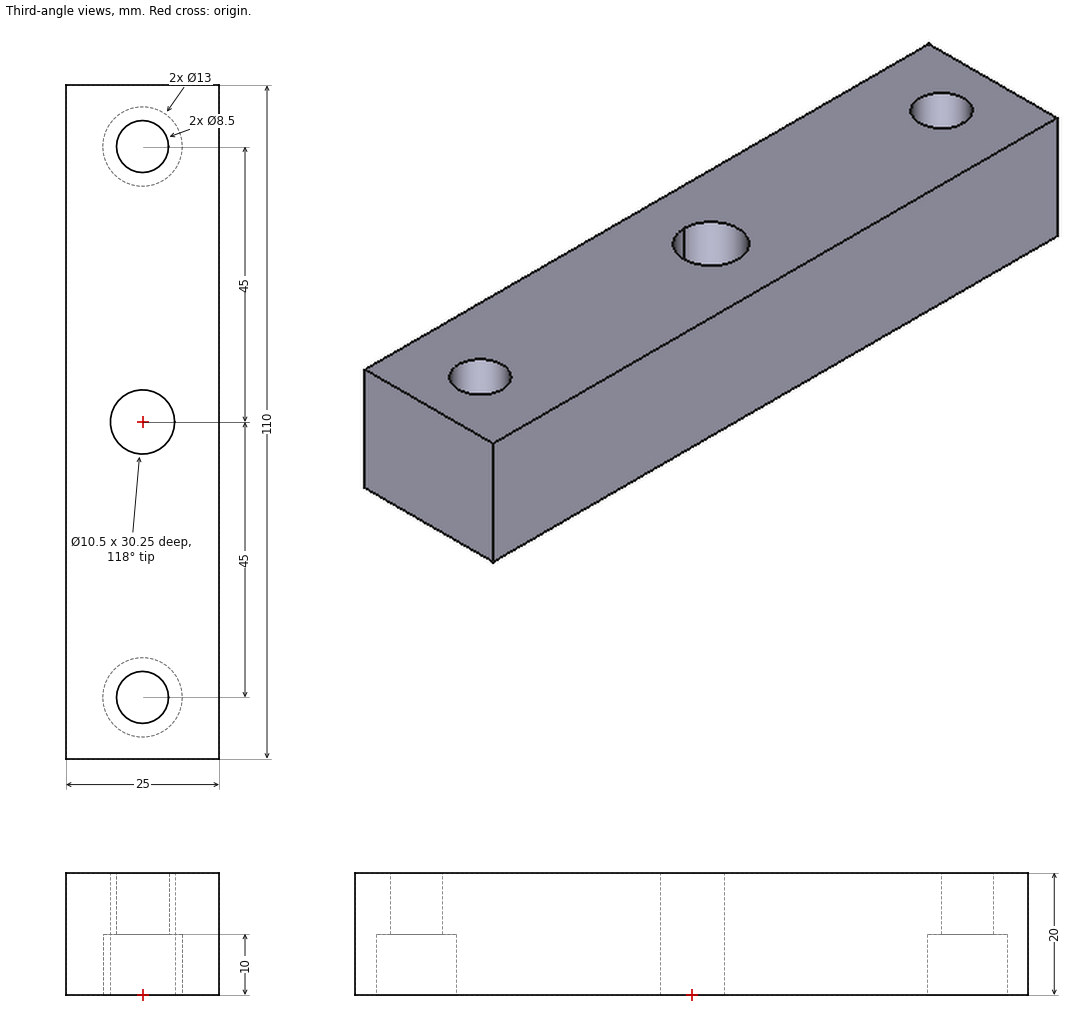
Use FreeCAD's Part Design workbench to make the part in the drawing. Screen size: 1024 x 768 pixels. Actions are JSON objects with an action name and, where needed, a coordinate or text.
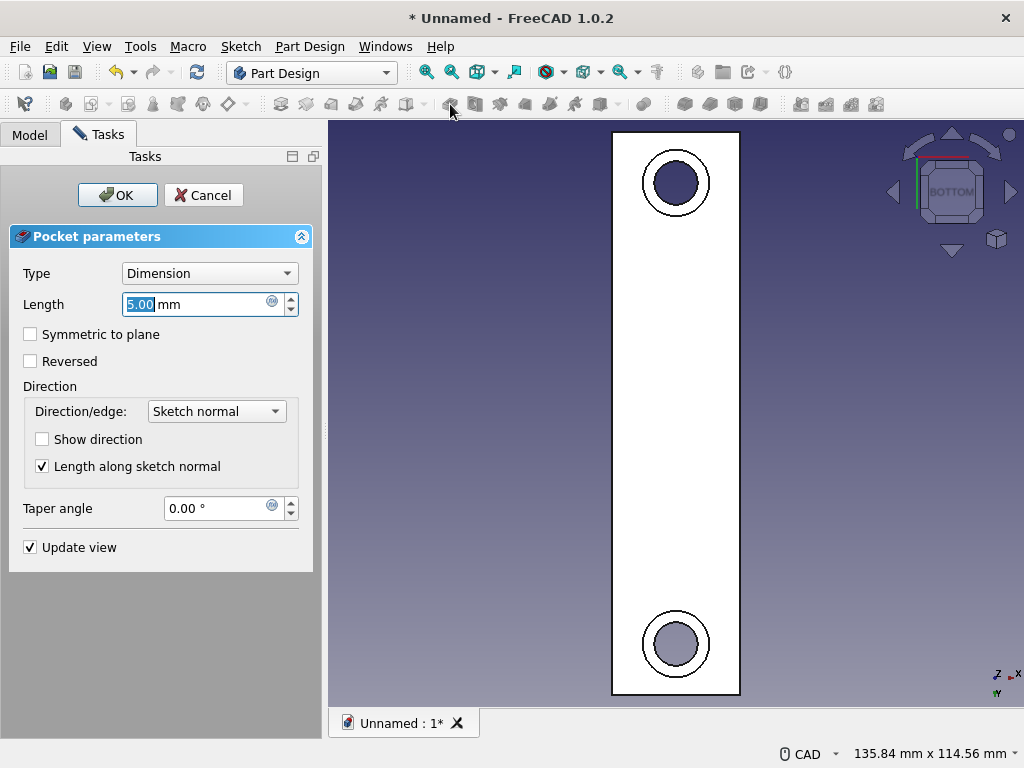
{"action": "type", "text": "10"}
{"action": "key", "text": "Tab"}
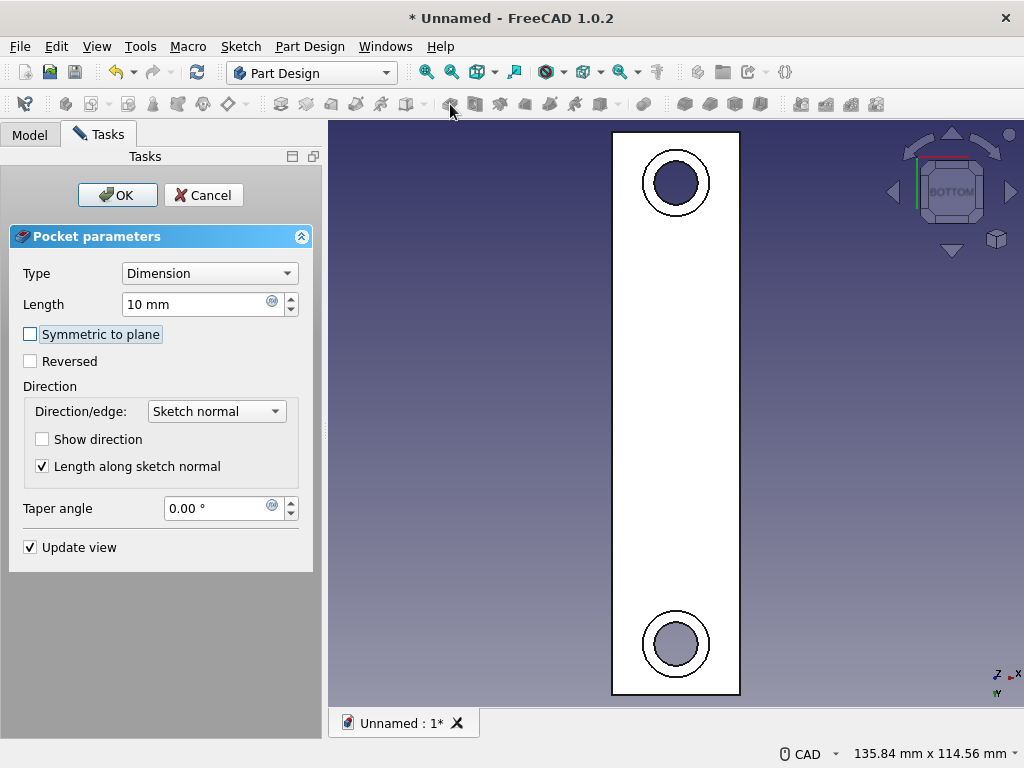
{"action": "left_click", "coordinate": [118, 195]}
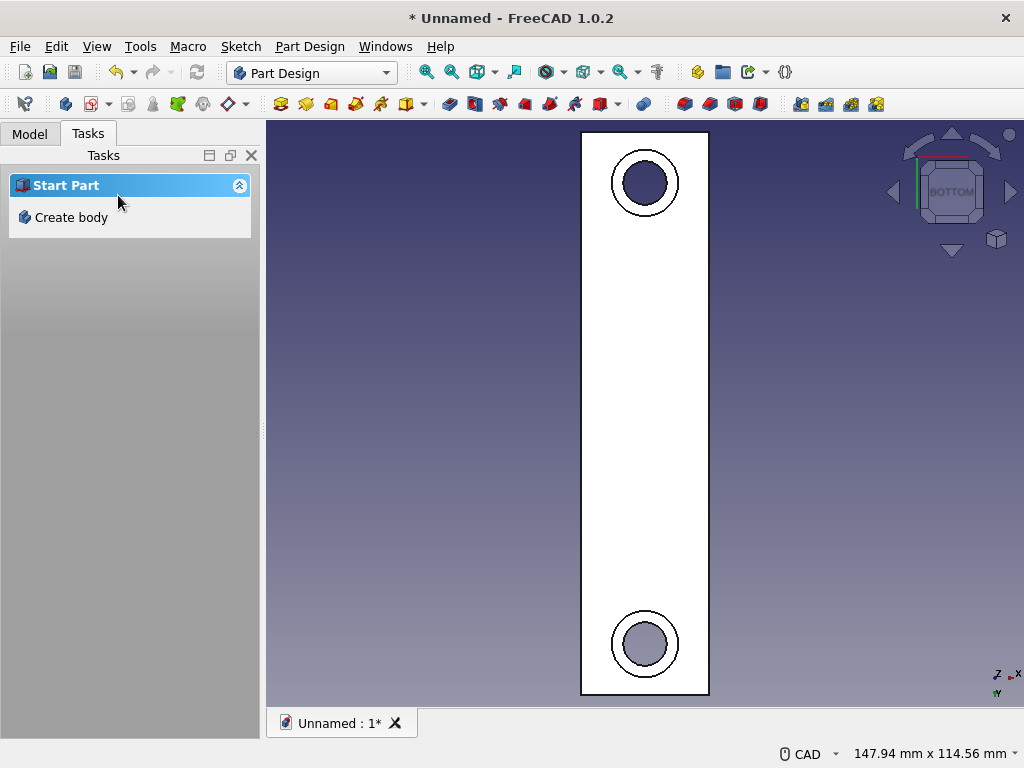
{"action": "left_click", "coordinate": [90, 104]}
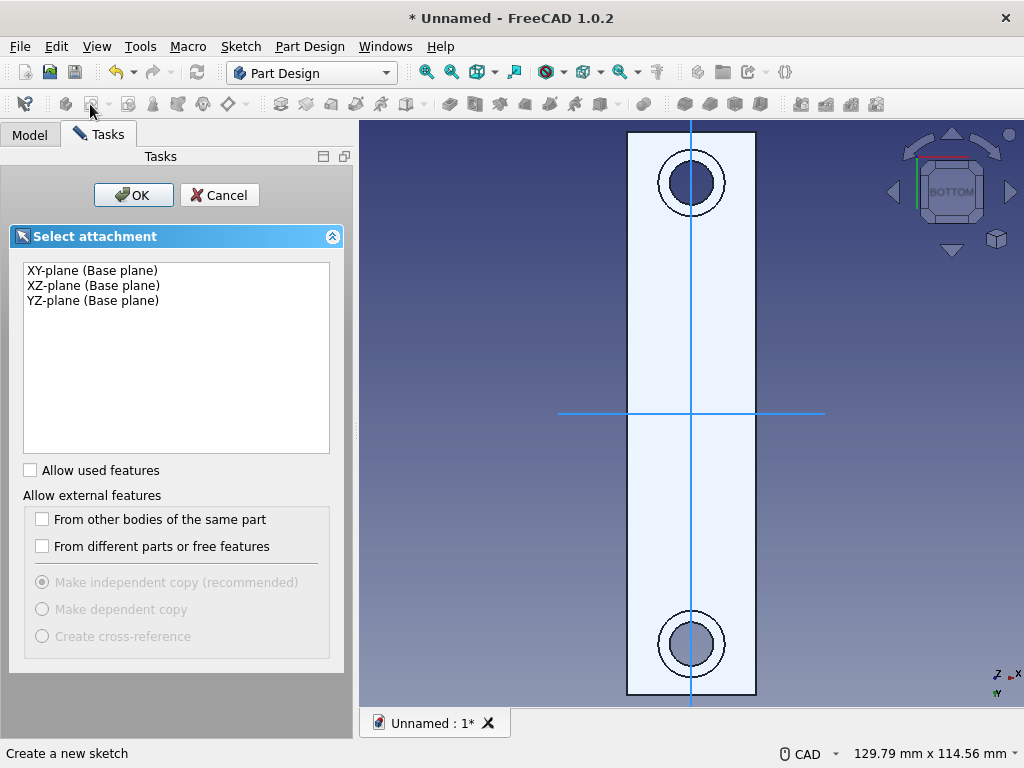
{"action": "left_click", "coordinate": [84, 270]}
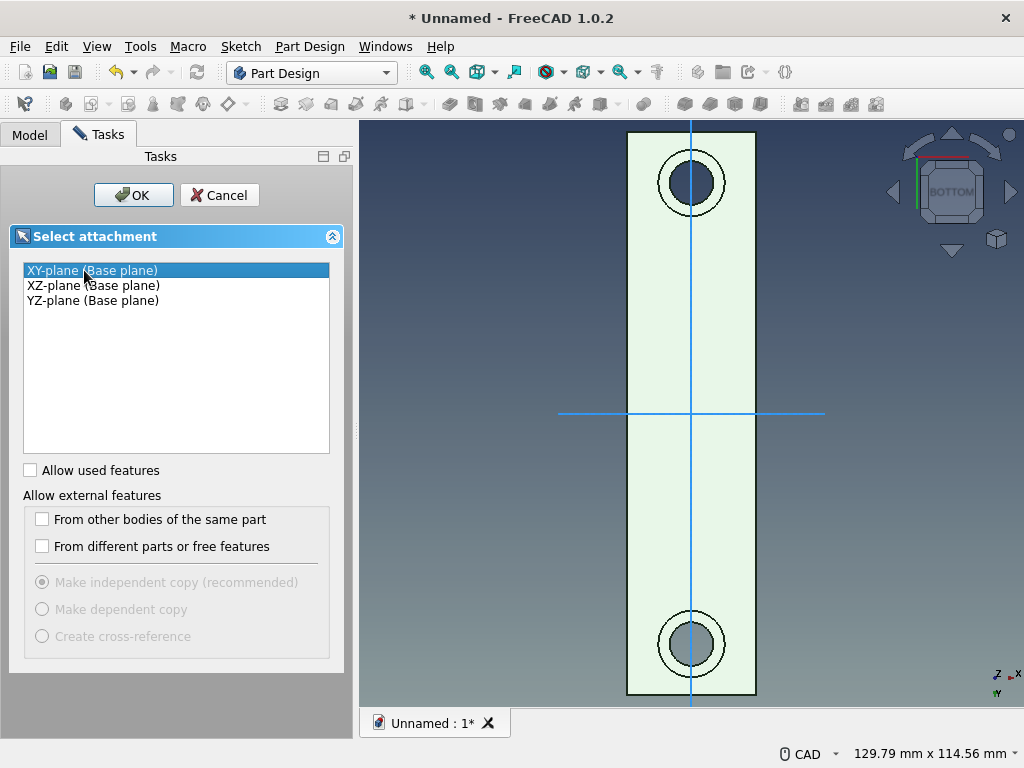
{"action": "left_click", "coordinate": [134, 195]}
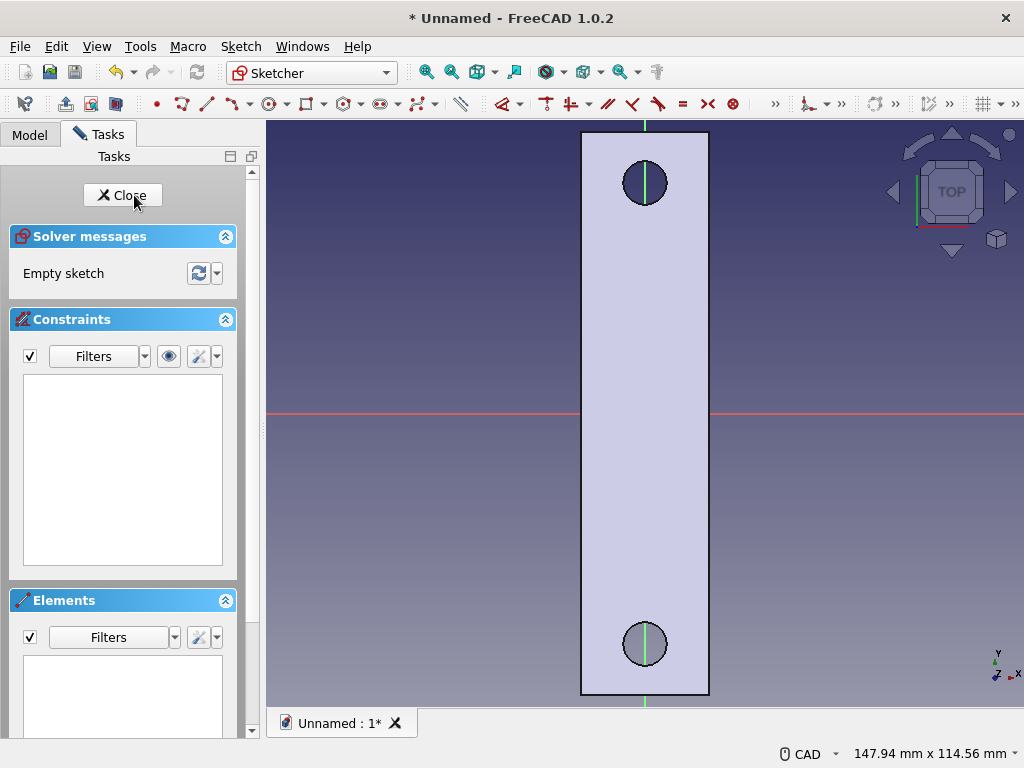
{"action": "key", "text": "q s"}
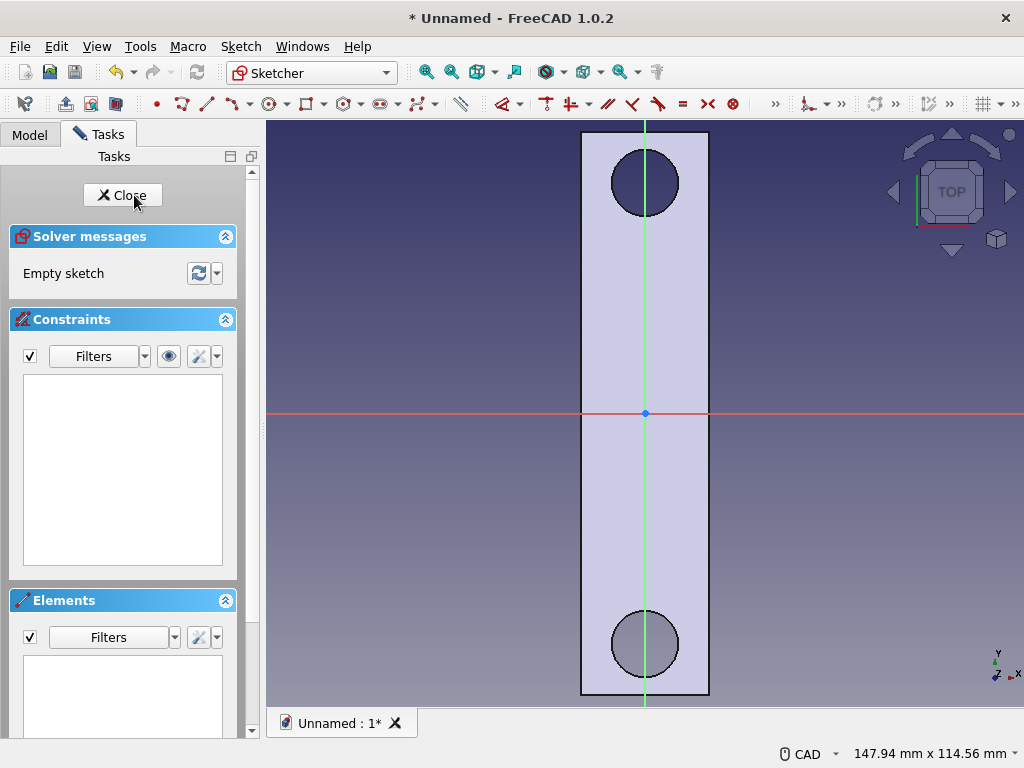
{"action": "scroll", "coordinate": [656, 413], "scroll_direction": "up", "scroll_amount": 10}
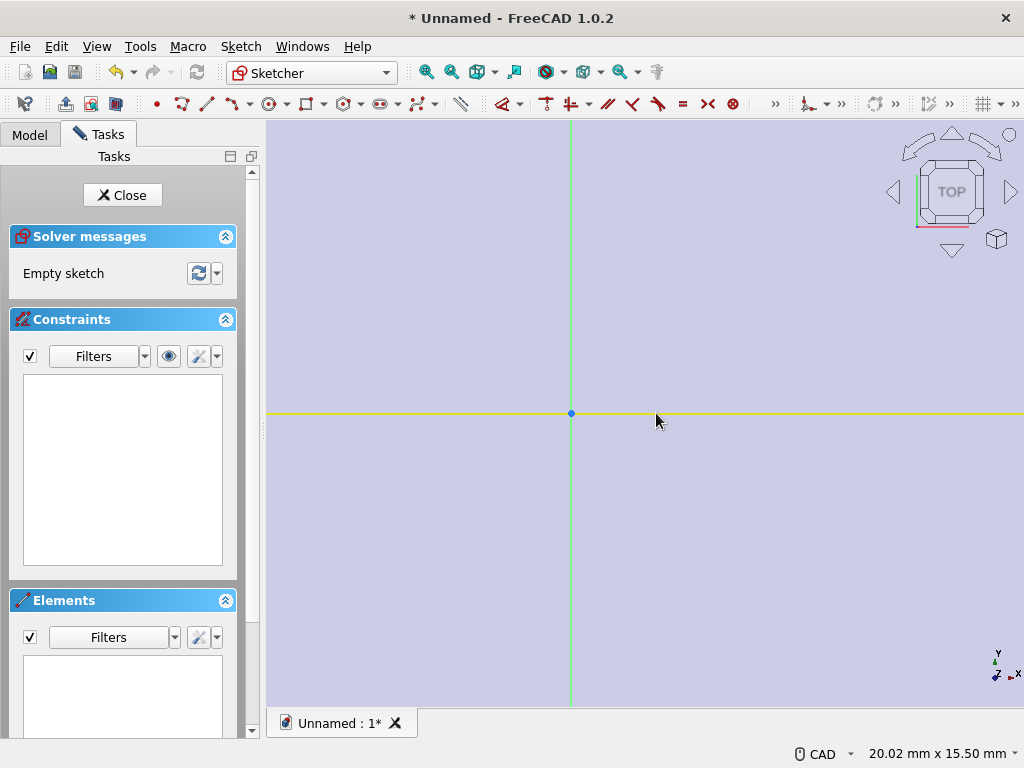
{"action": "left_click", "coordinate": [268, 104]}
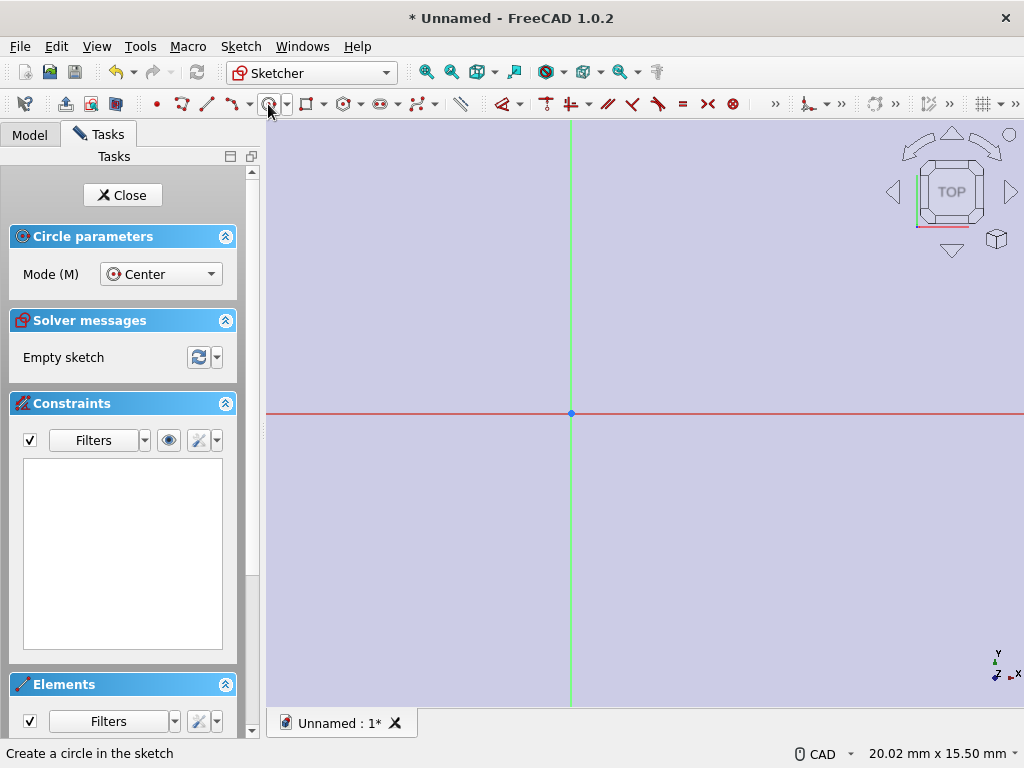
{"action": "left_click", "coordinate": [571, 413]}
{"action": "left_click", "coordinate": [712, 273]}
{"action": "key", "text": "Escape"}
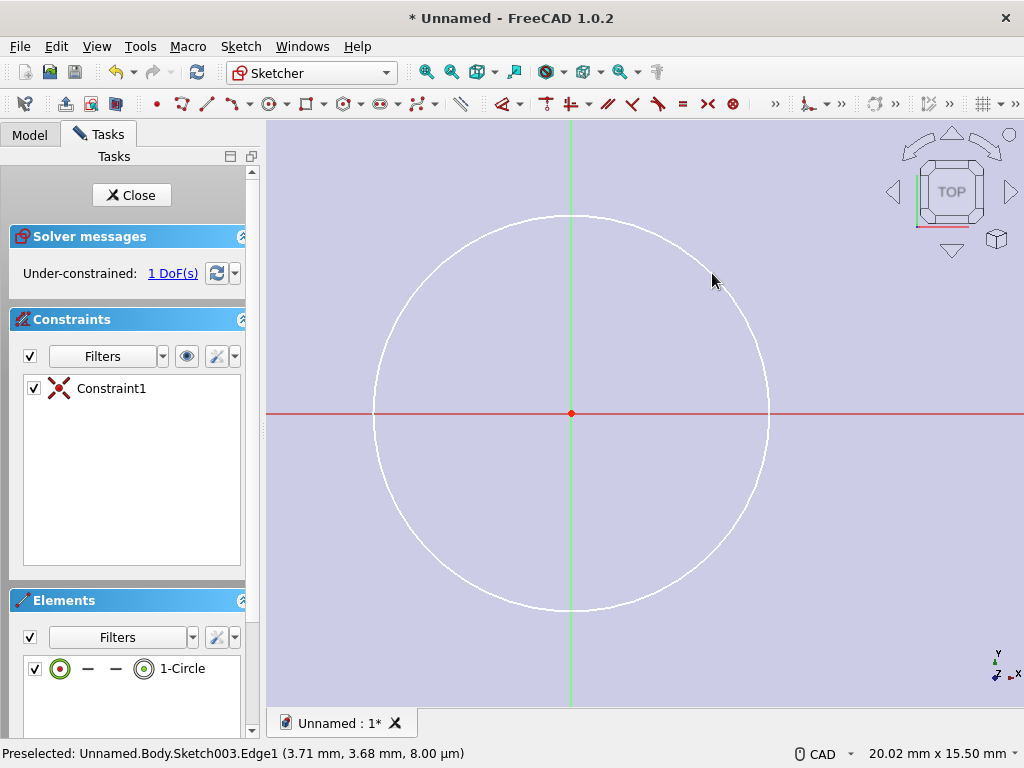
{"action": "left_click", "coordinate": [502, 104]}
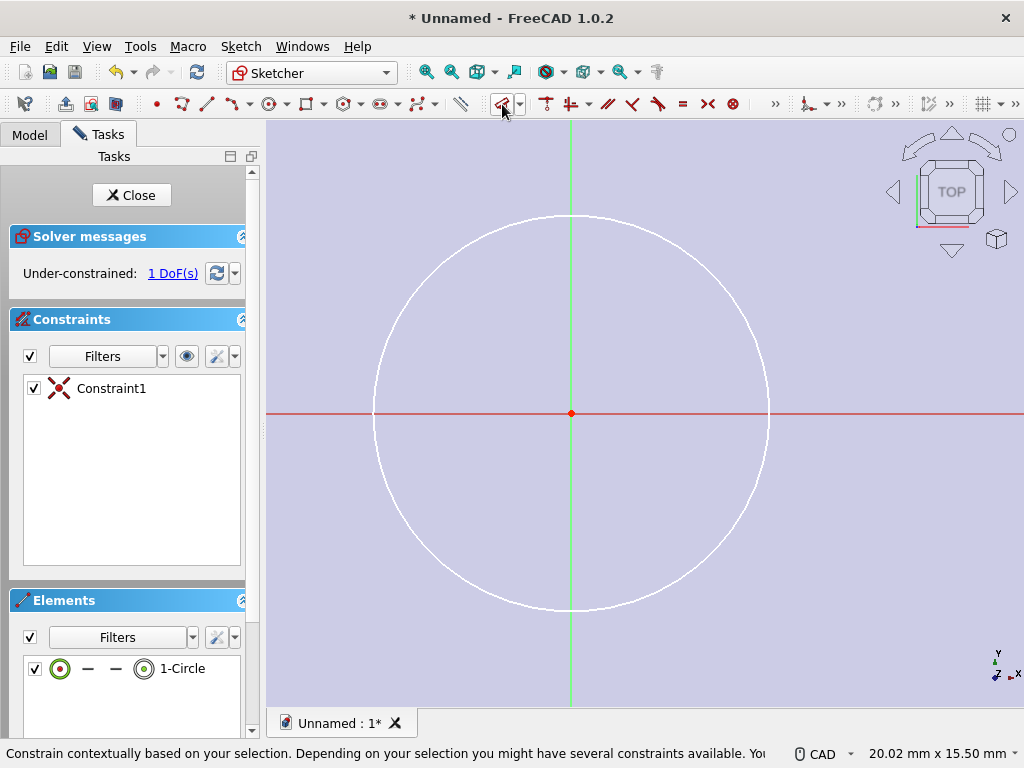
{"action": "left_click", "coordinate": [711, 273]}
{"action": "left_click", "coordinate": [734, 250]}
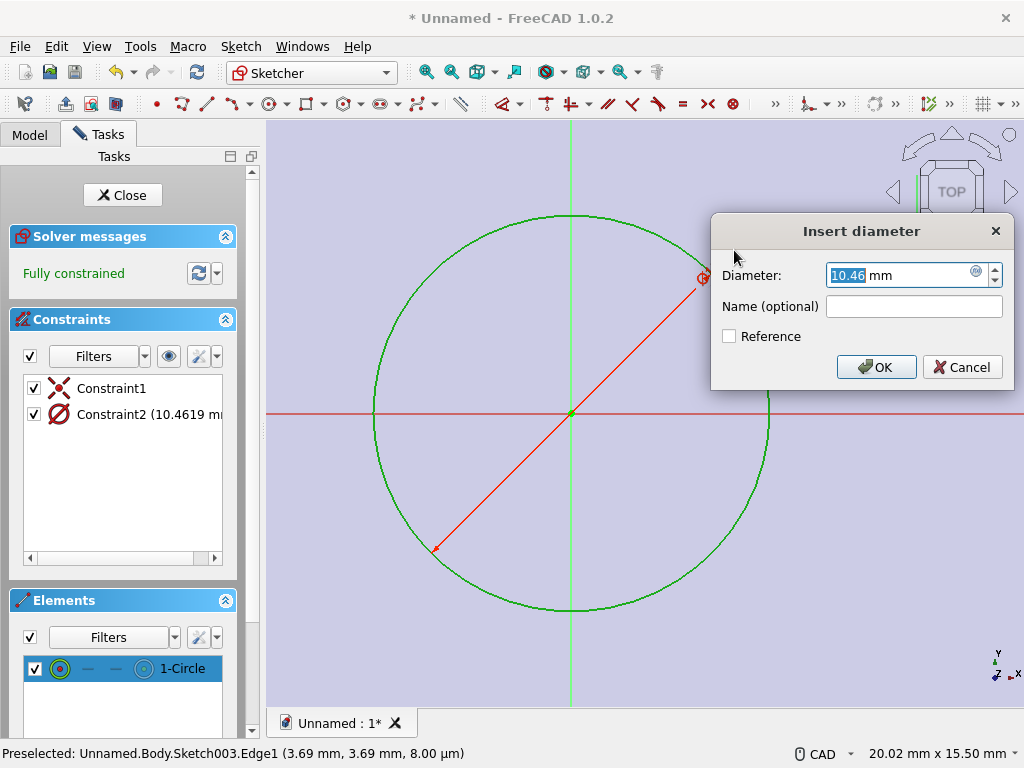
{"action": "type", "text": "10.5"}
{"action": "key", "text": "Return"}
{"action": "key", "text": "Escape"}